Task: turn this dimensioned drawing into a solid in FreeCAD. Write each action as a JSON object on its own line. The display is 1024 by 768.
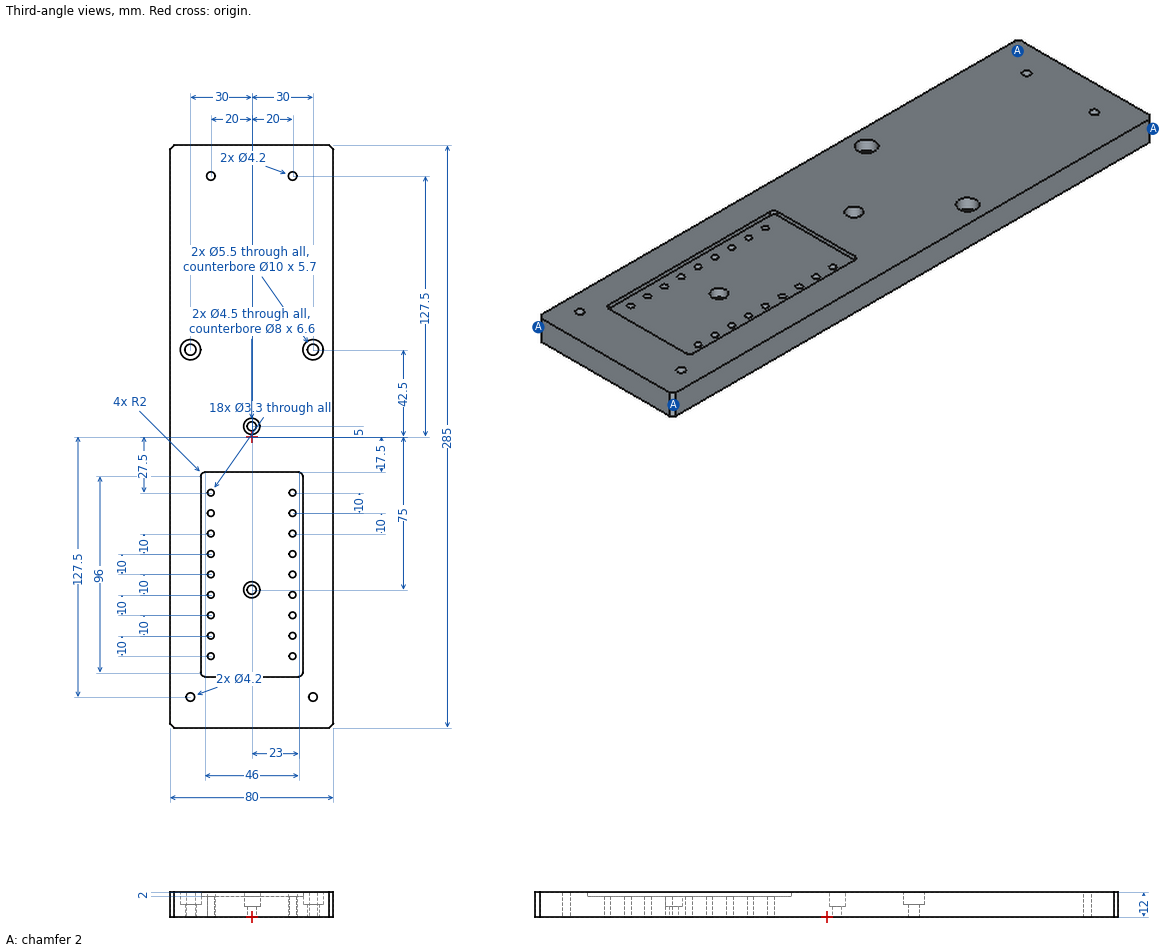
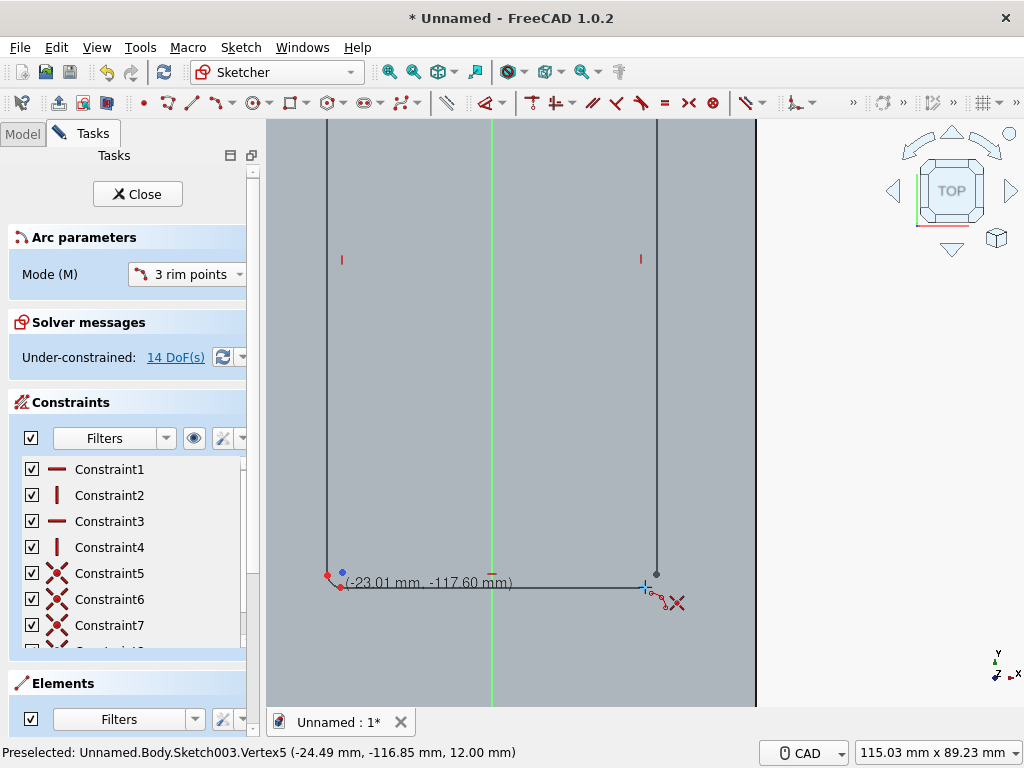
{"action": "left_click", "coordinate": [644, 588]}
{"action": "left_click", "coordinate": [657, 575]}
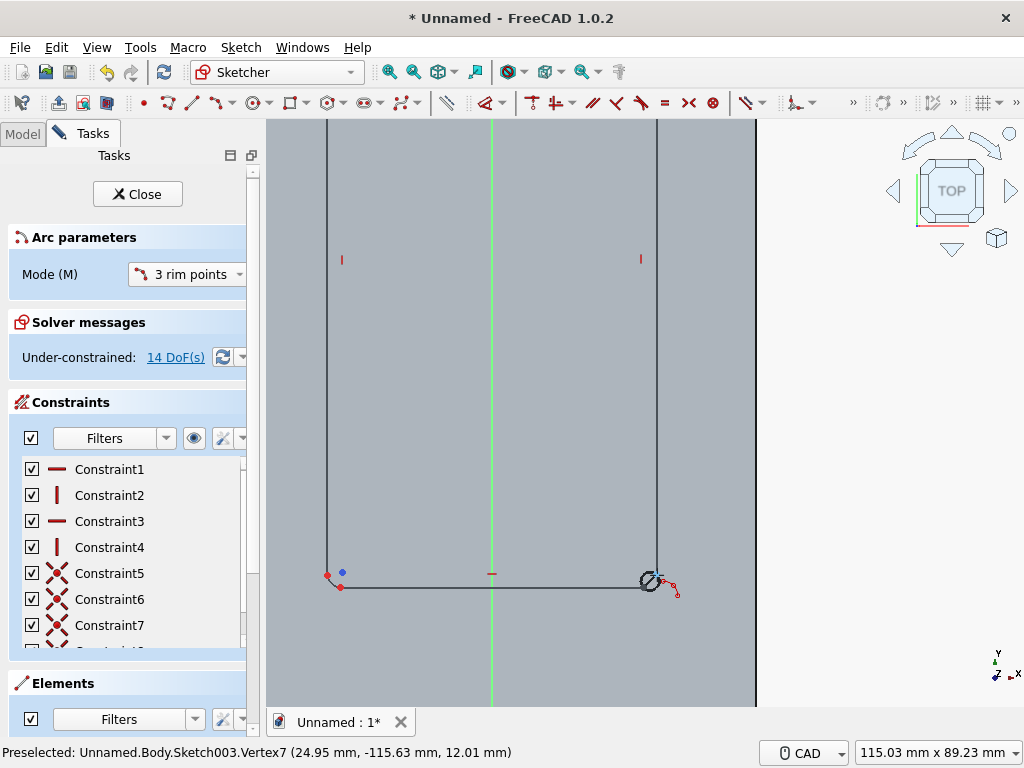
{"action": "scroll", "coordinate": [653, 583], "scroll_direction": "up", "scroll_amount": 8}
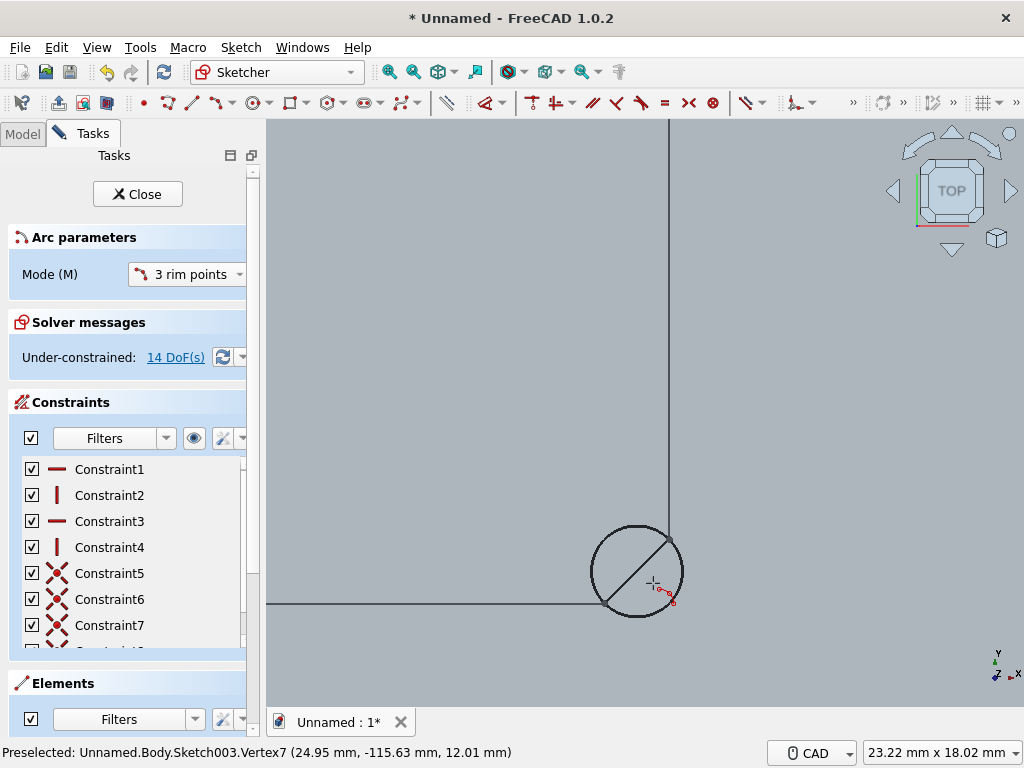
{"action": "left_click", "coordinate": [652, 581]}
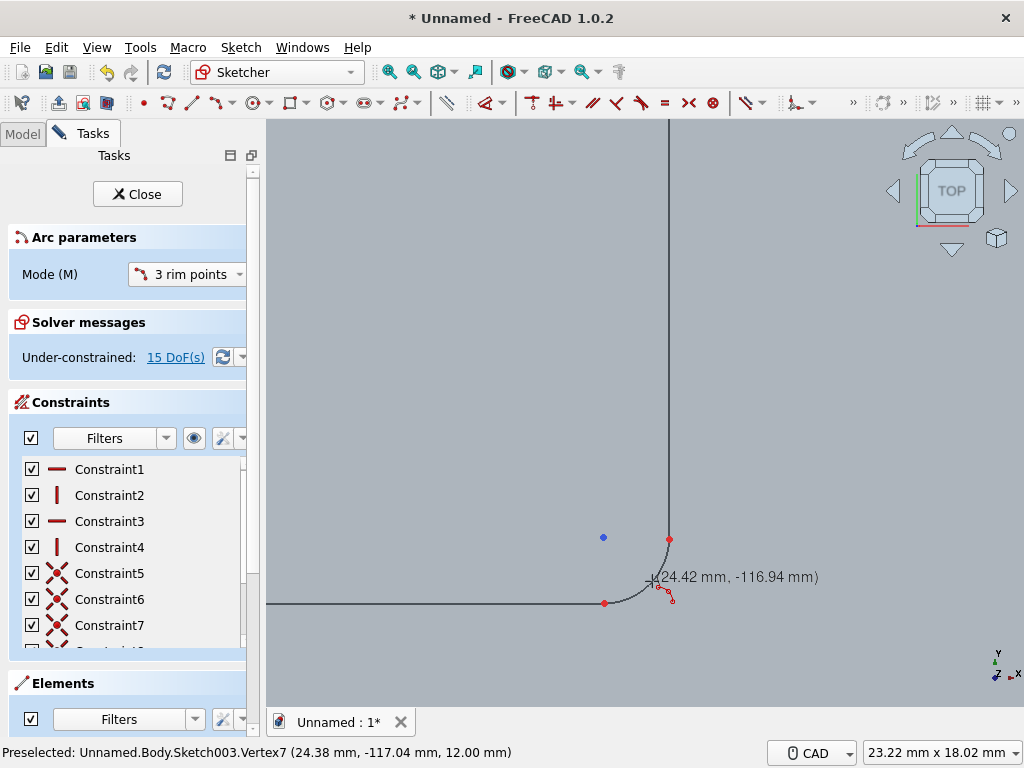
{"action": "scroll", "coordinate": [648, 586], "scroll_direction": "down", "scroll_amount": 12}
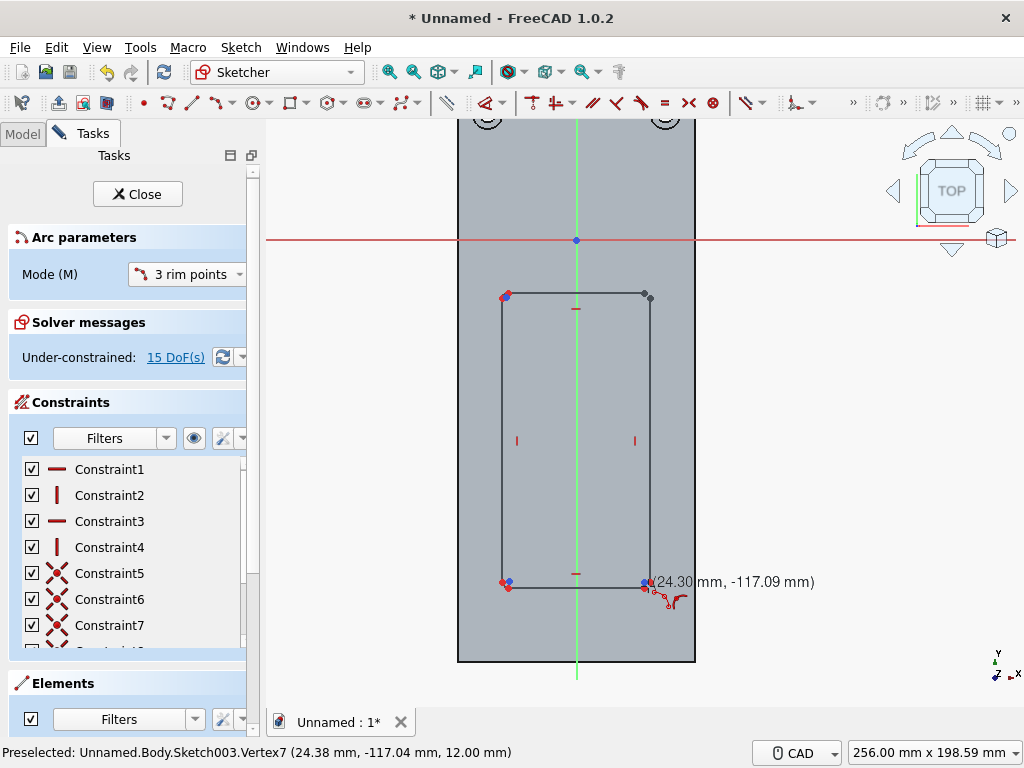
{"action": "scroll", "coordinate": [651, 298], "scroll_direction": "up", "scroll_amount": 4}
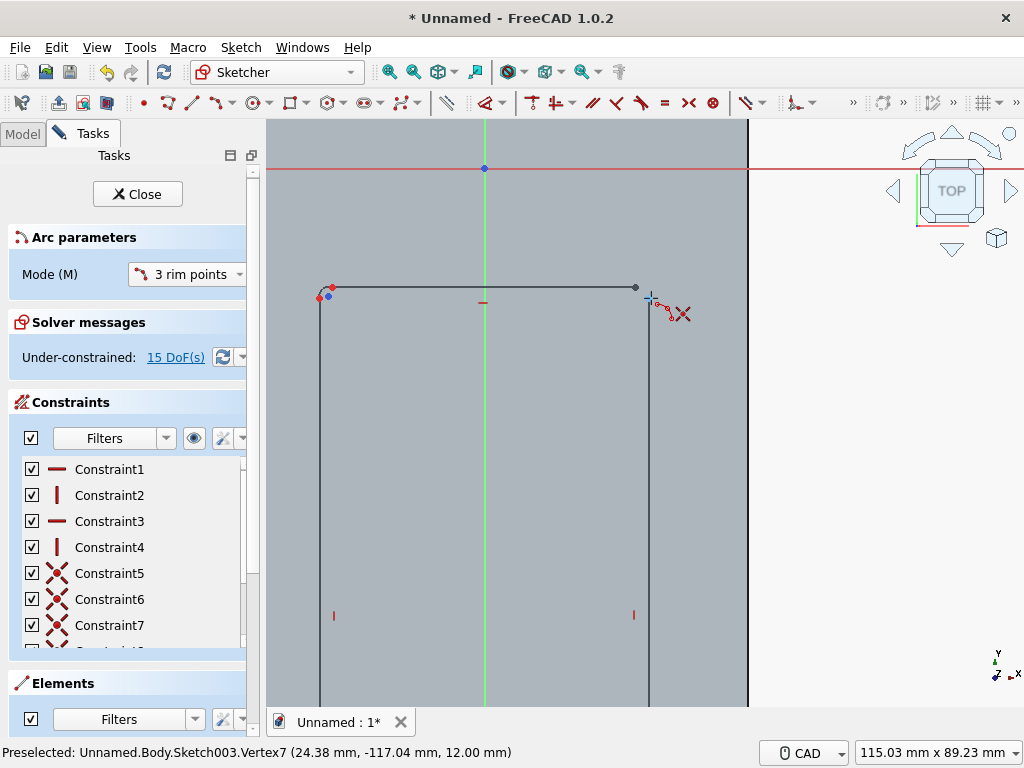
{"action": "left_click", "coordinate": [649, 299]}
{"action": "left_click", "coordinate": [635, 287]}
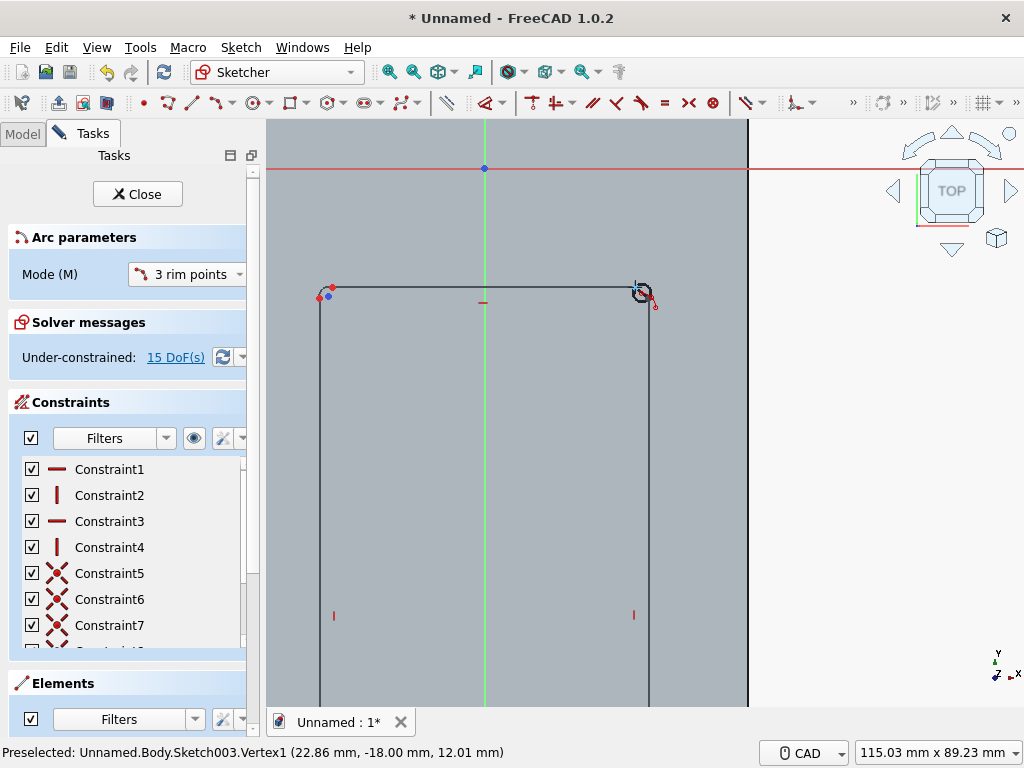
{"action": "scroll", "coordinate": [645, 288], "scroll_direction": "up", "scroll_amount": 8}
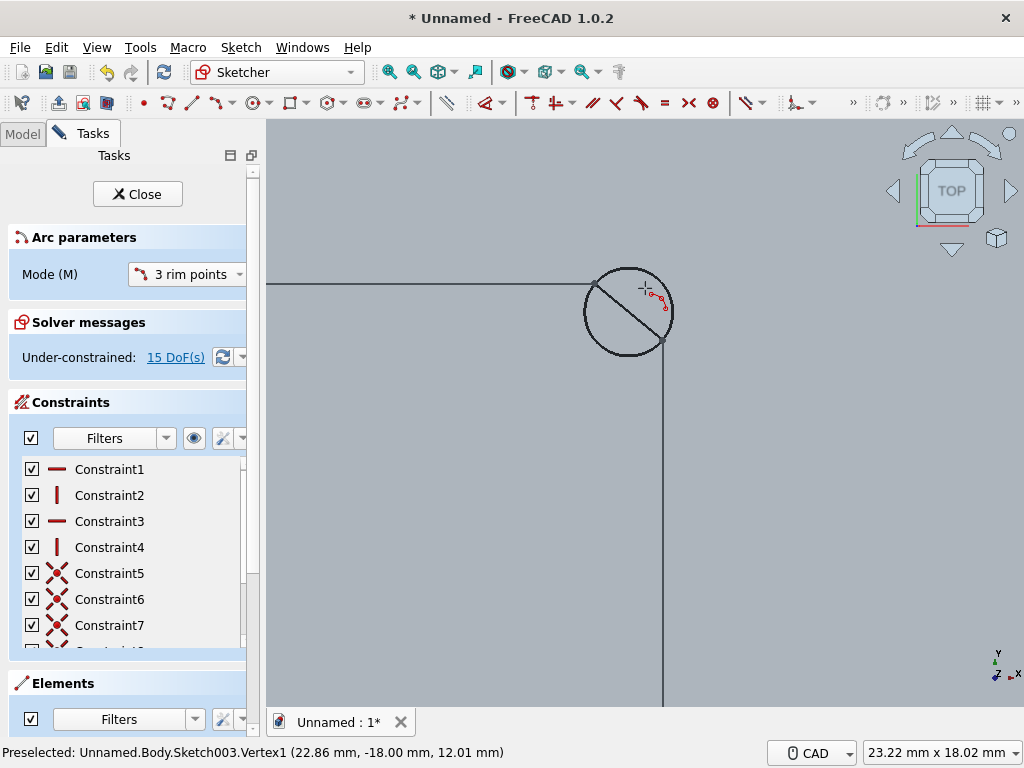
{"action": "left_click", "coordinate": [645, 287]}
{"action": "key", "text": "Escape"}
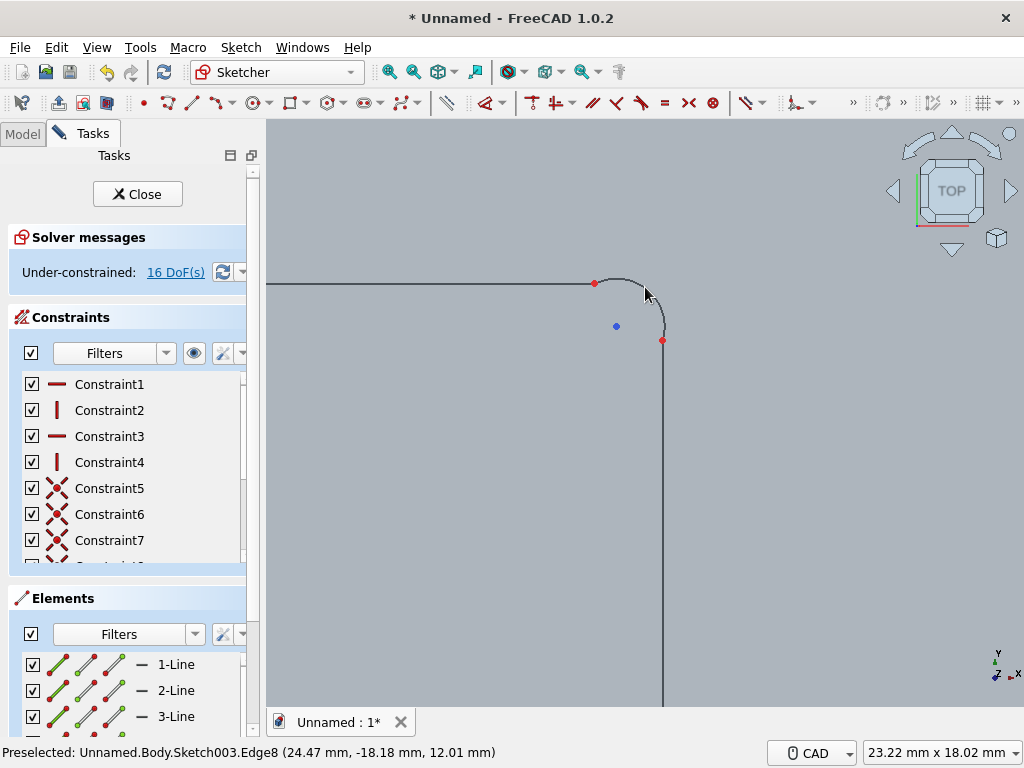
{"action": "scroll", "coordinate": [649, 293], "scroll_direction": "down", "scroll_amount": 12}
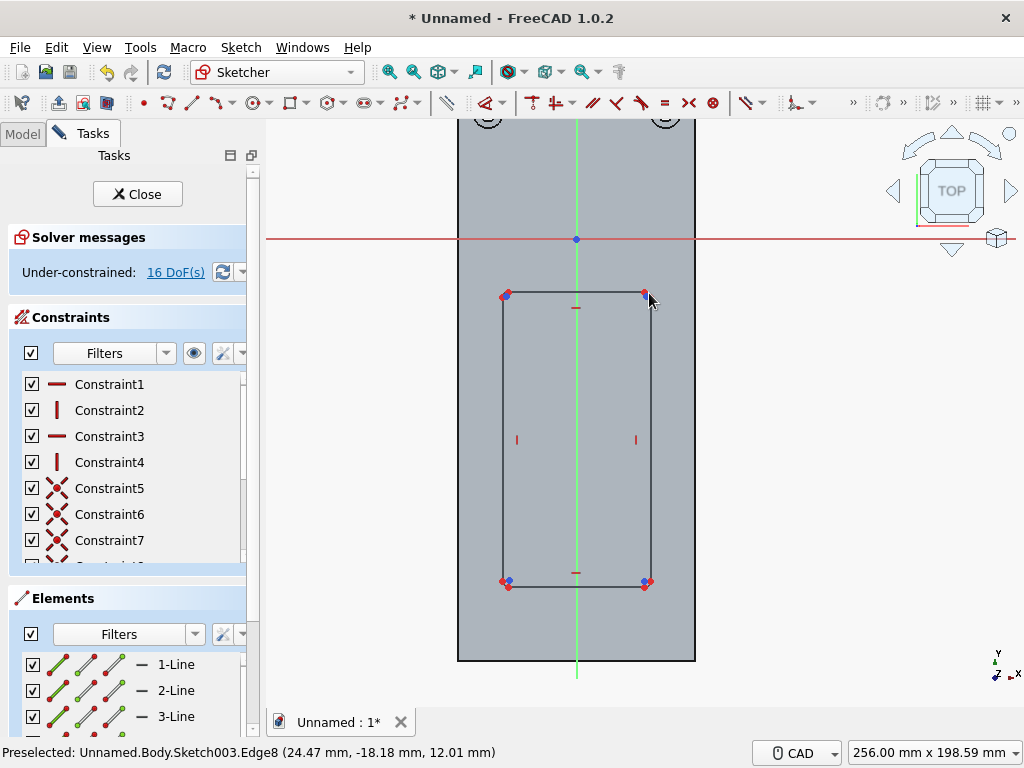
{"action": "left_click", "coordinate": [617, 292]}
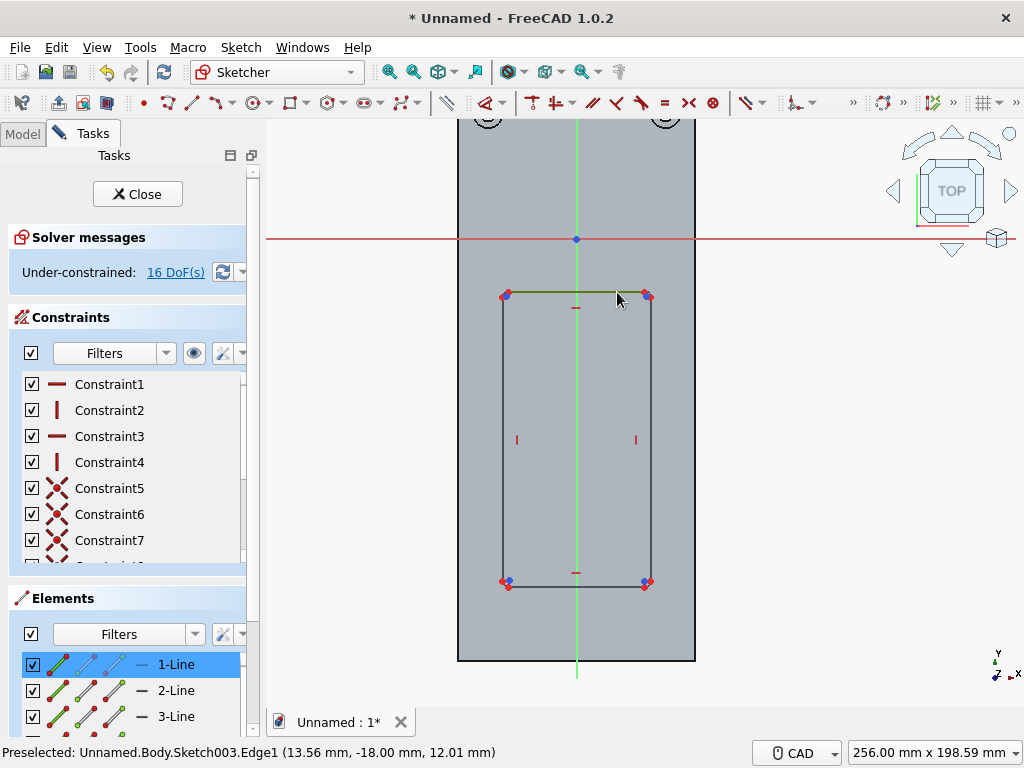
{"action": "scroll", "coordinate": [504, 293], "scroll_direction": "up", "scroll_amount": 6}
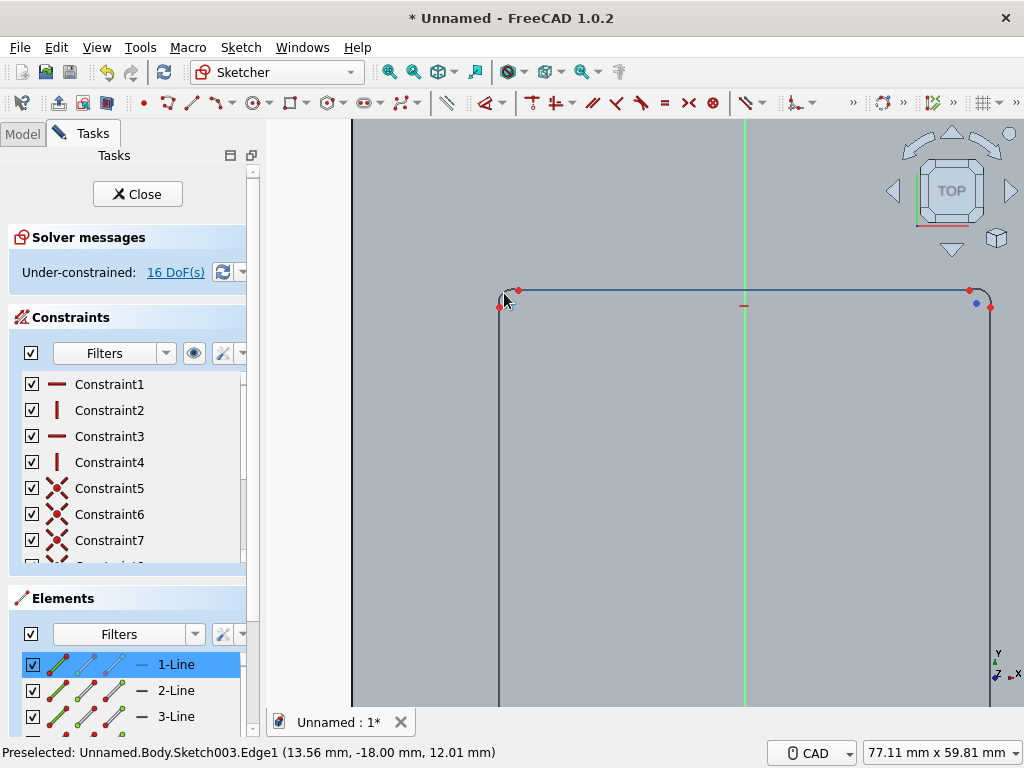
{"action": "left_click", "coordinate": [503, 293]}